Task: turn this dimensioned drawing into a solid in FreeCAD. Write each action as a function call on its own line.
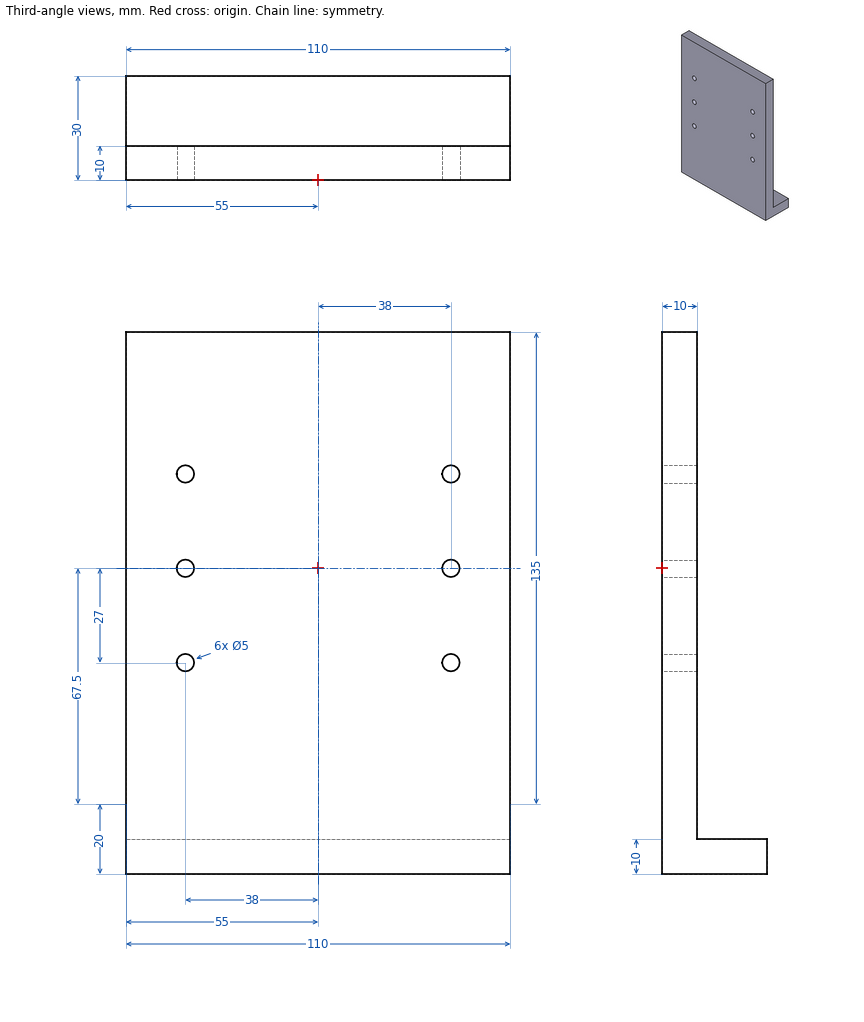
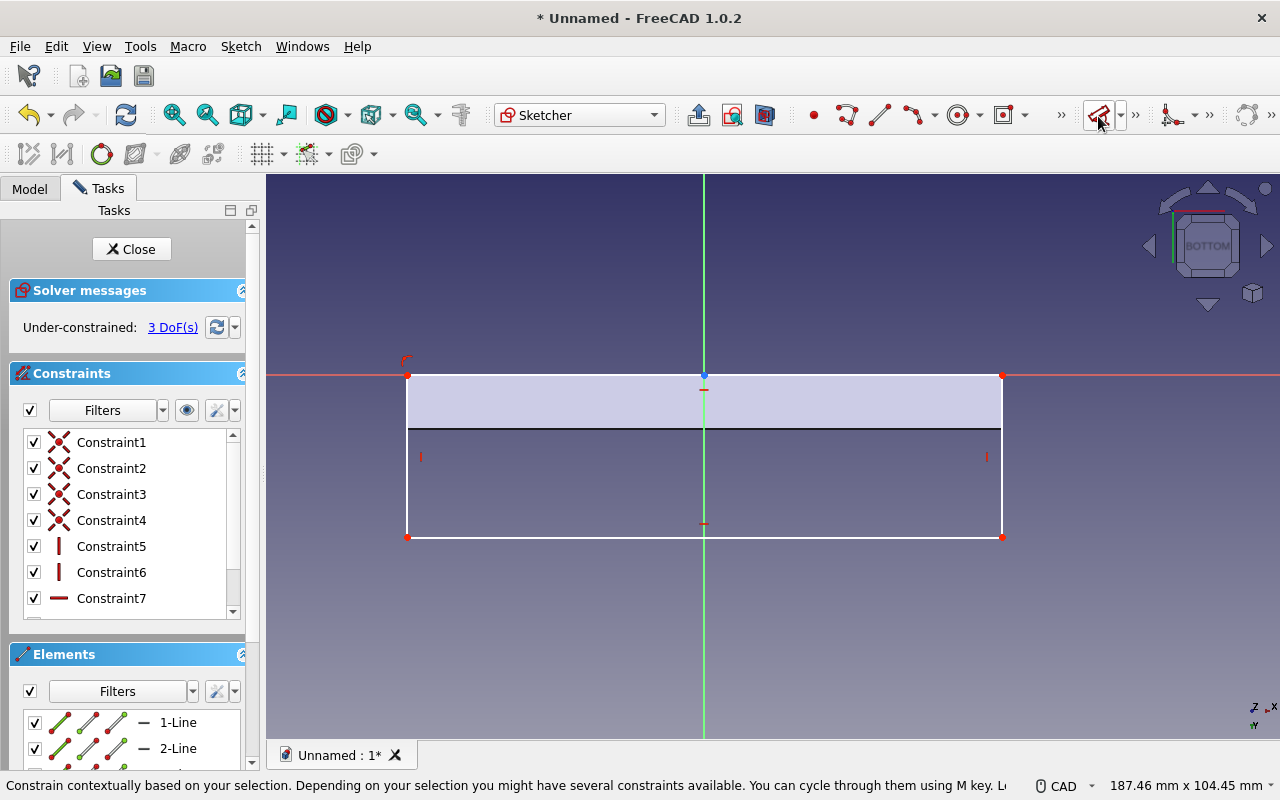
click(407, 424)
click(373, 457)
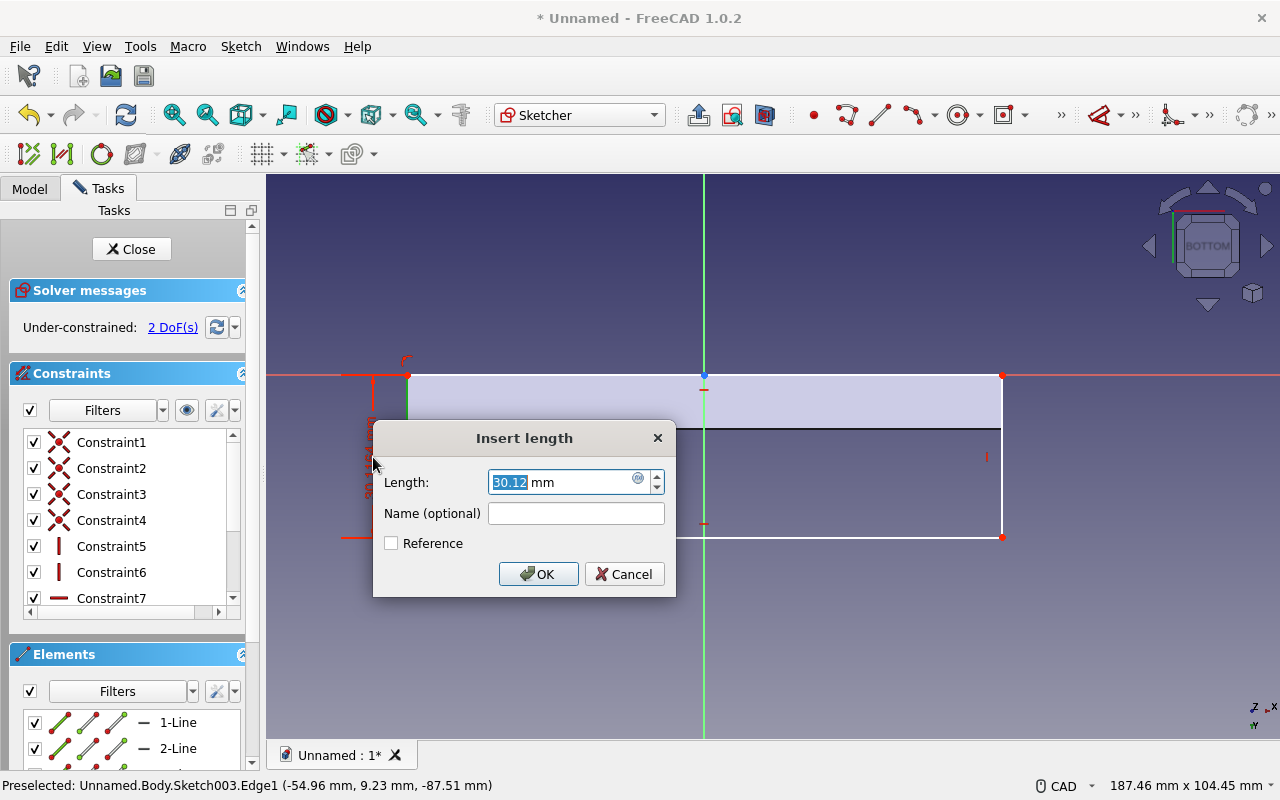
text(30)
key(Return)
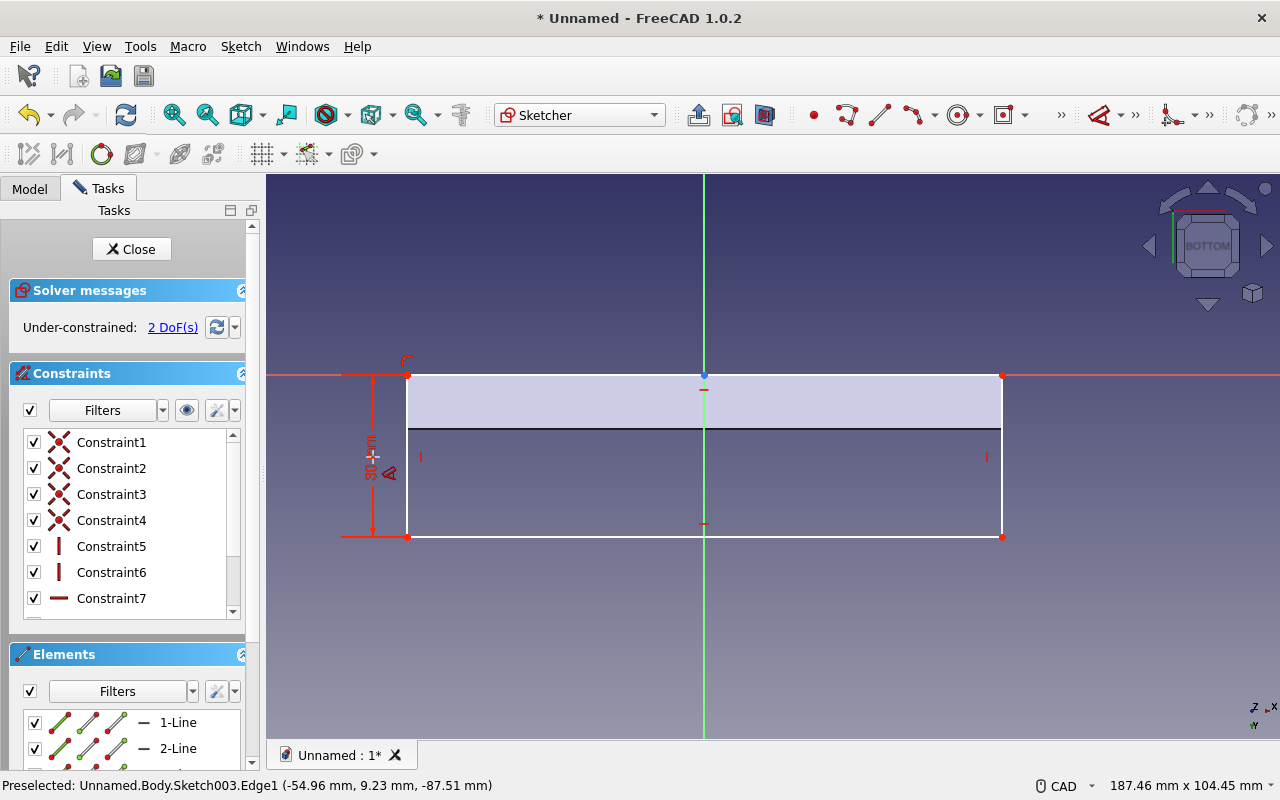
click(585, 537)
click(568, 571)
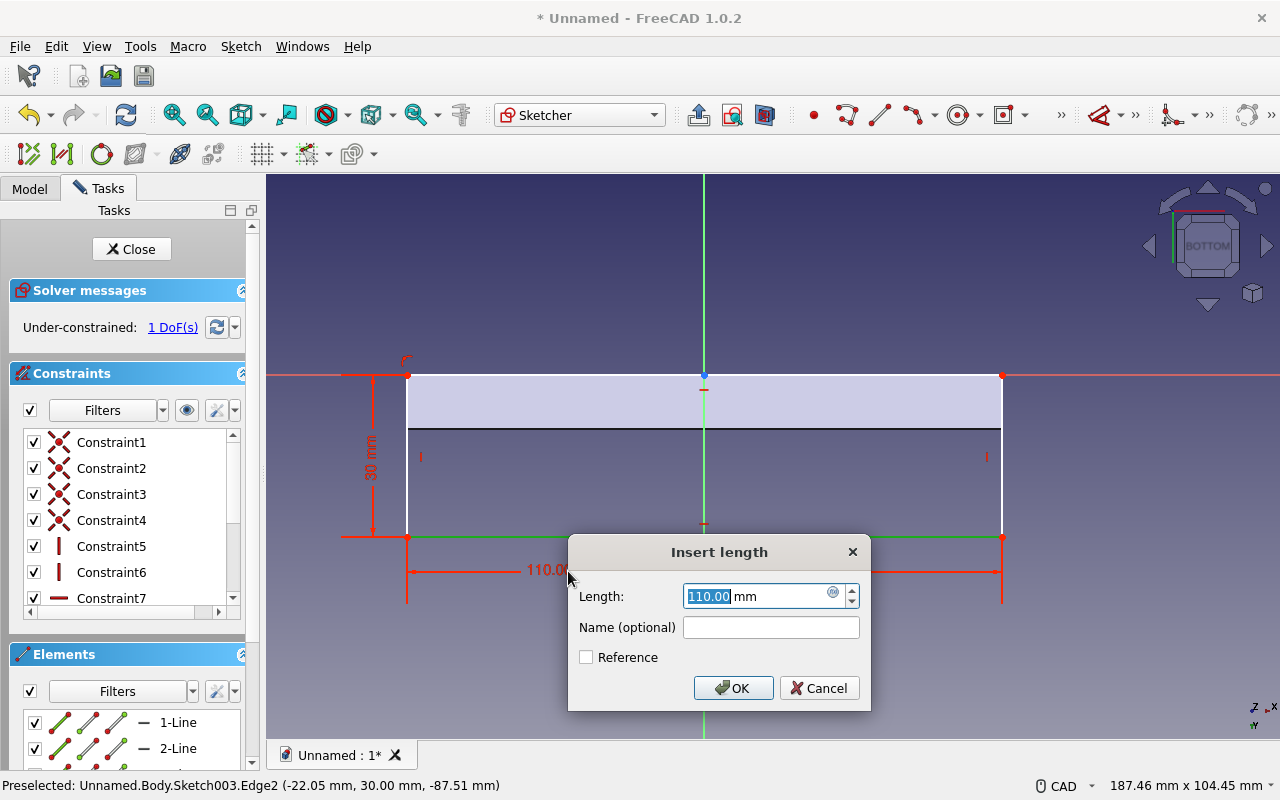
text(110)
key(Return)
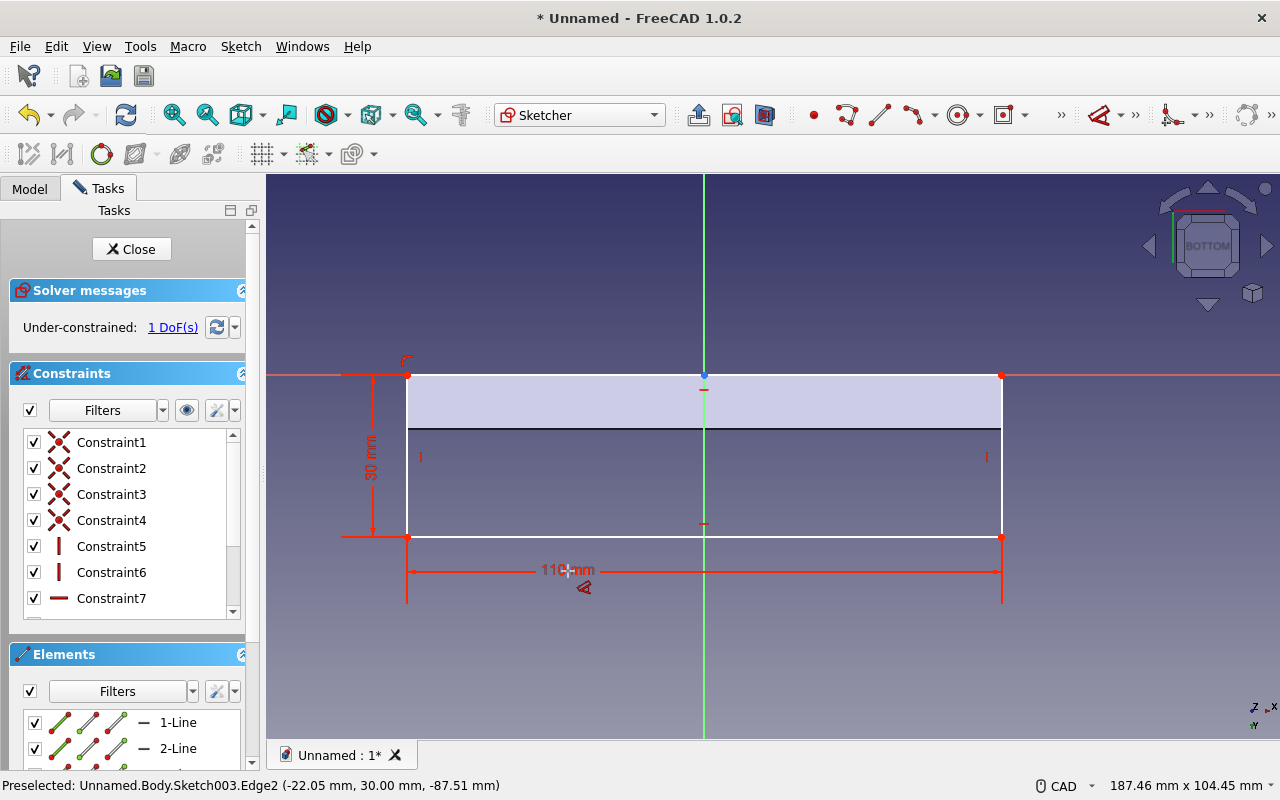
click(407, 375)
click(556, 341)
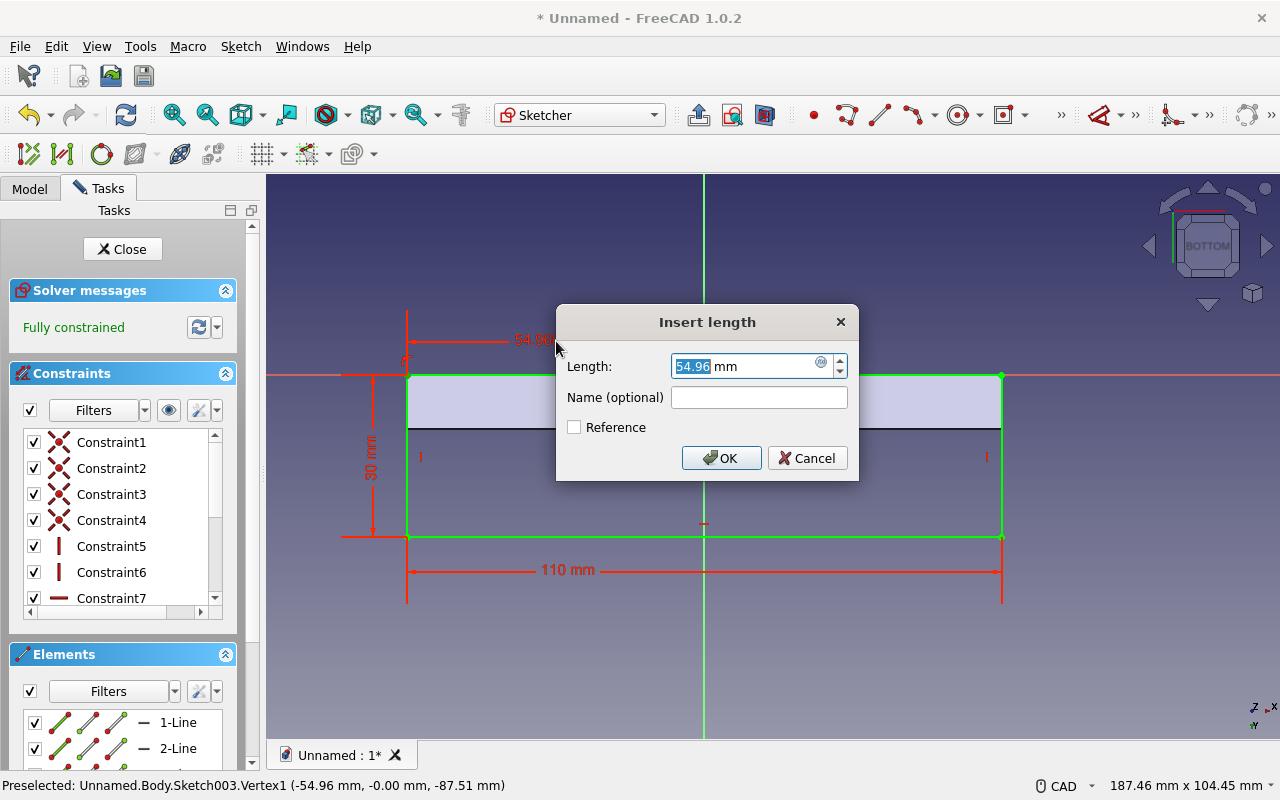
text(55)
key(Return)
key(Escape)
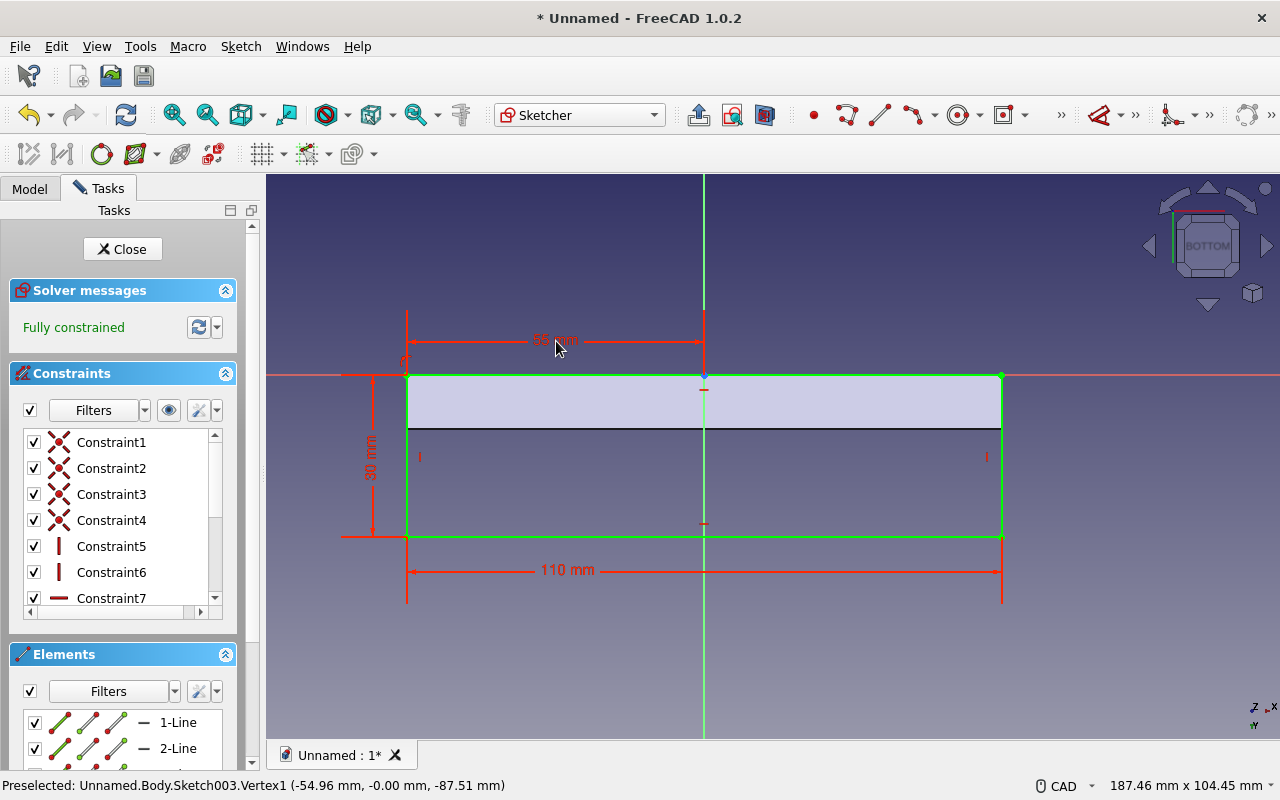
click(123, 249)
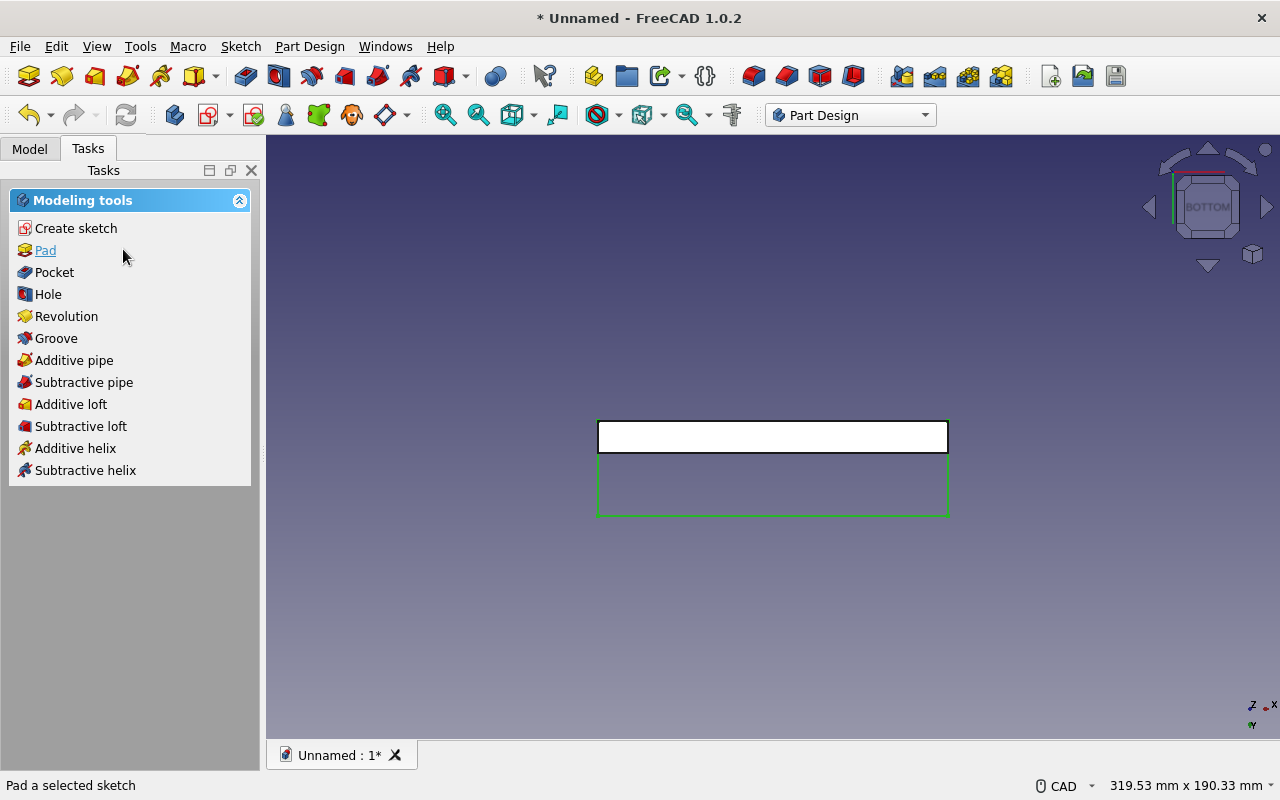
click(29, 76)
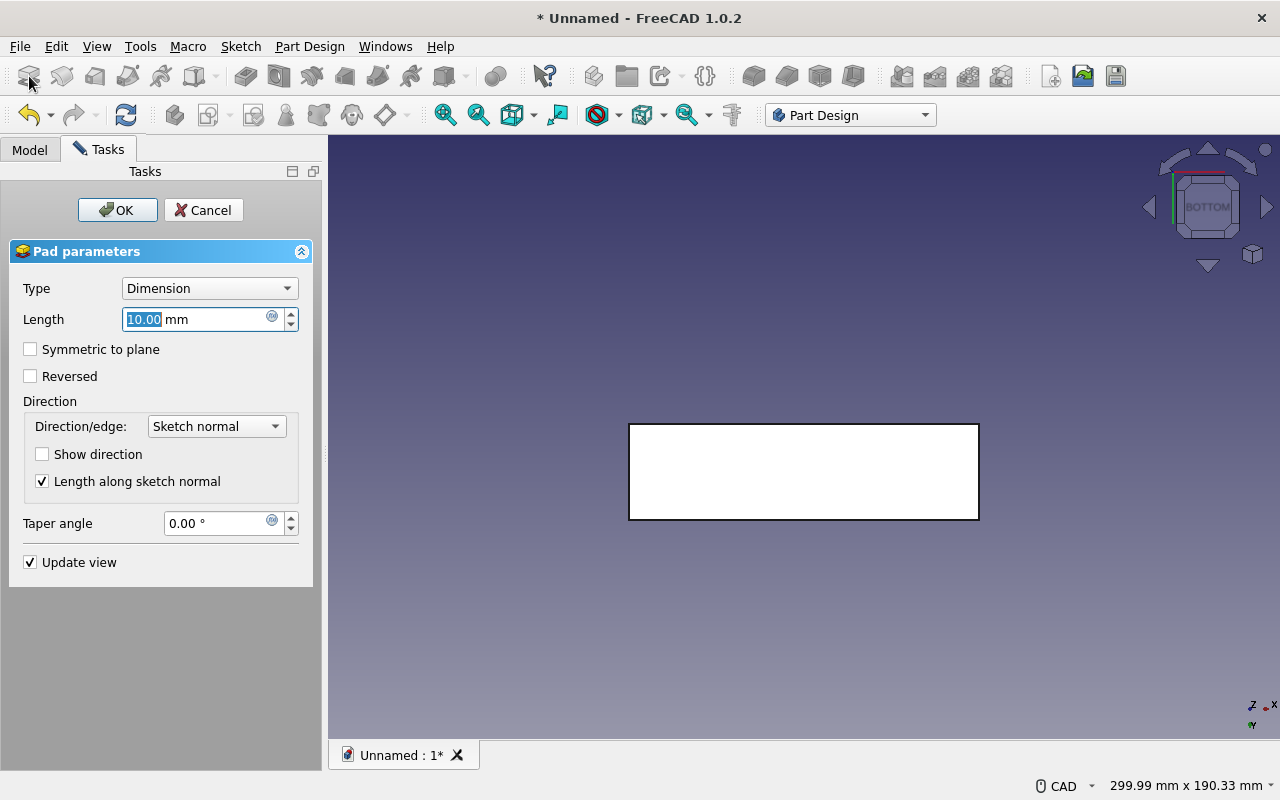
text(10)
key(Tab)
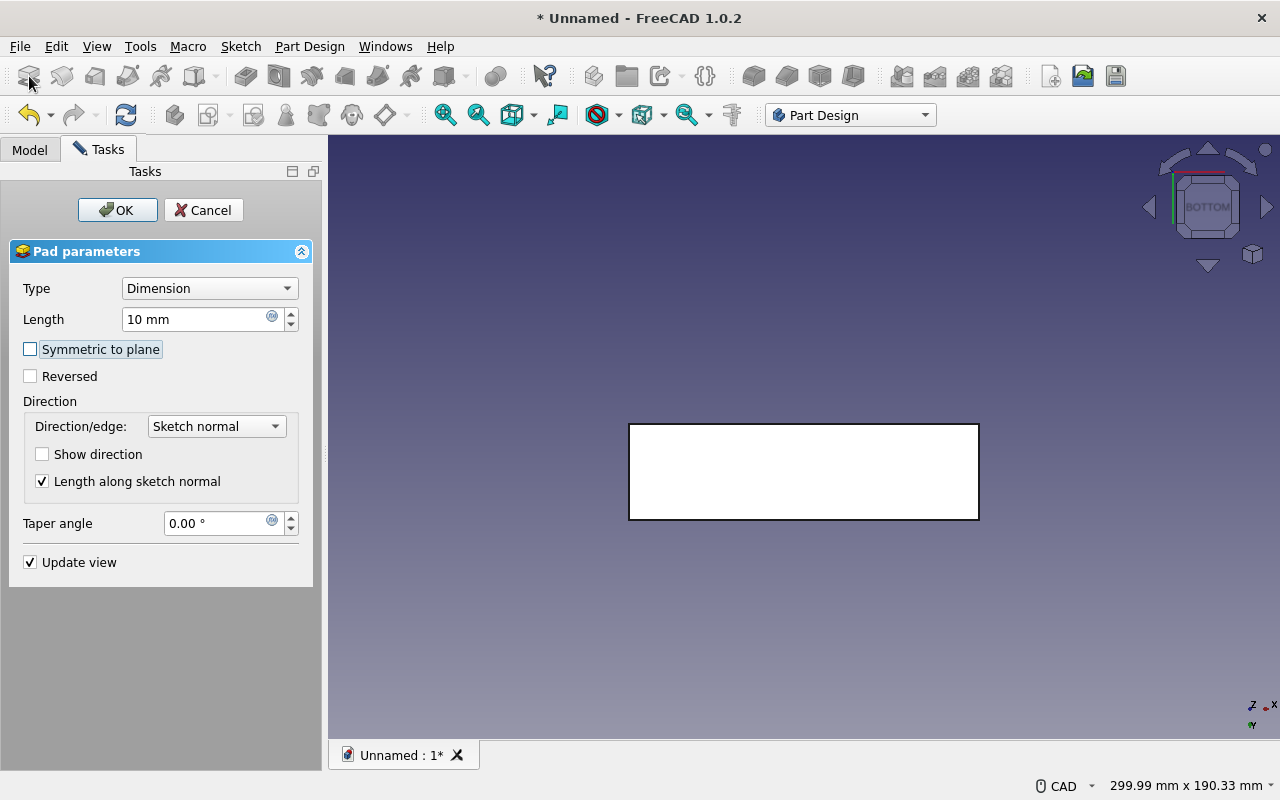
click(31, 376)